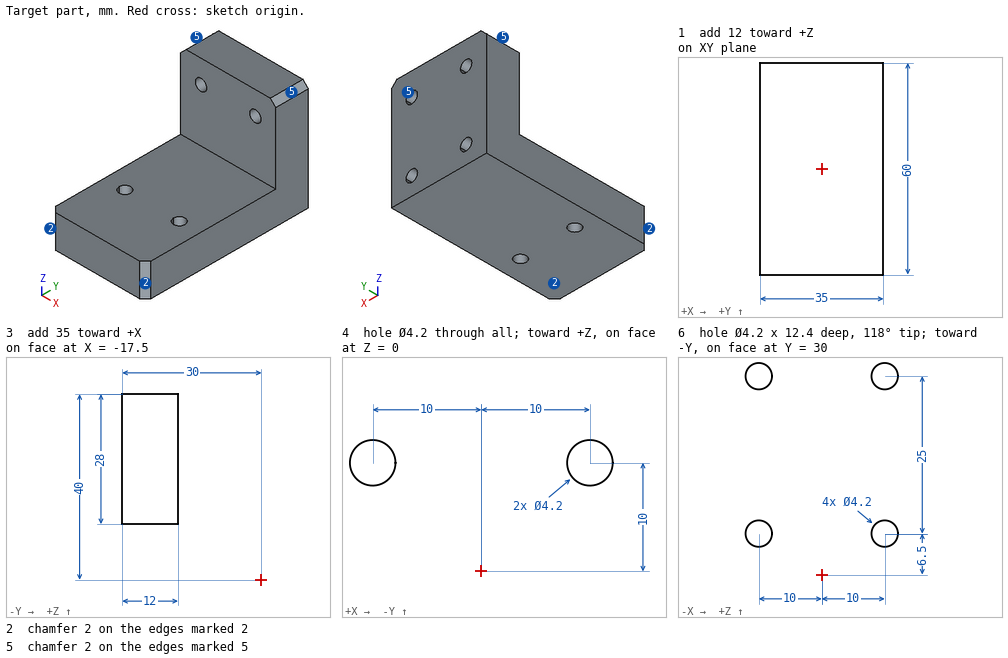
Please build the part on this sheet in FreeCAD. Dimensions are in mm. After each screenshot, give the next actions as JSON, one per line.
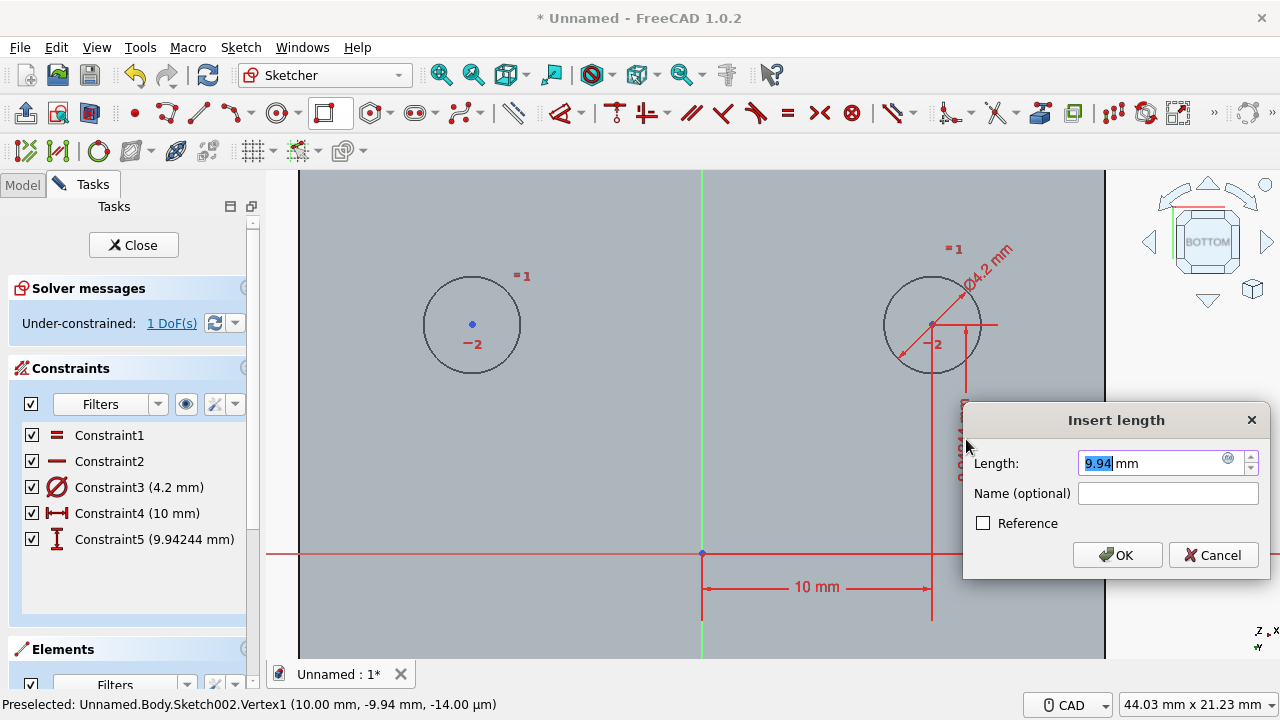
{"action": "type", "text": "10"}
{"action": "key", "text": "Return"}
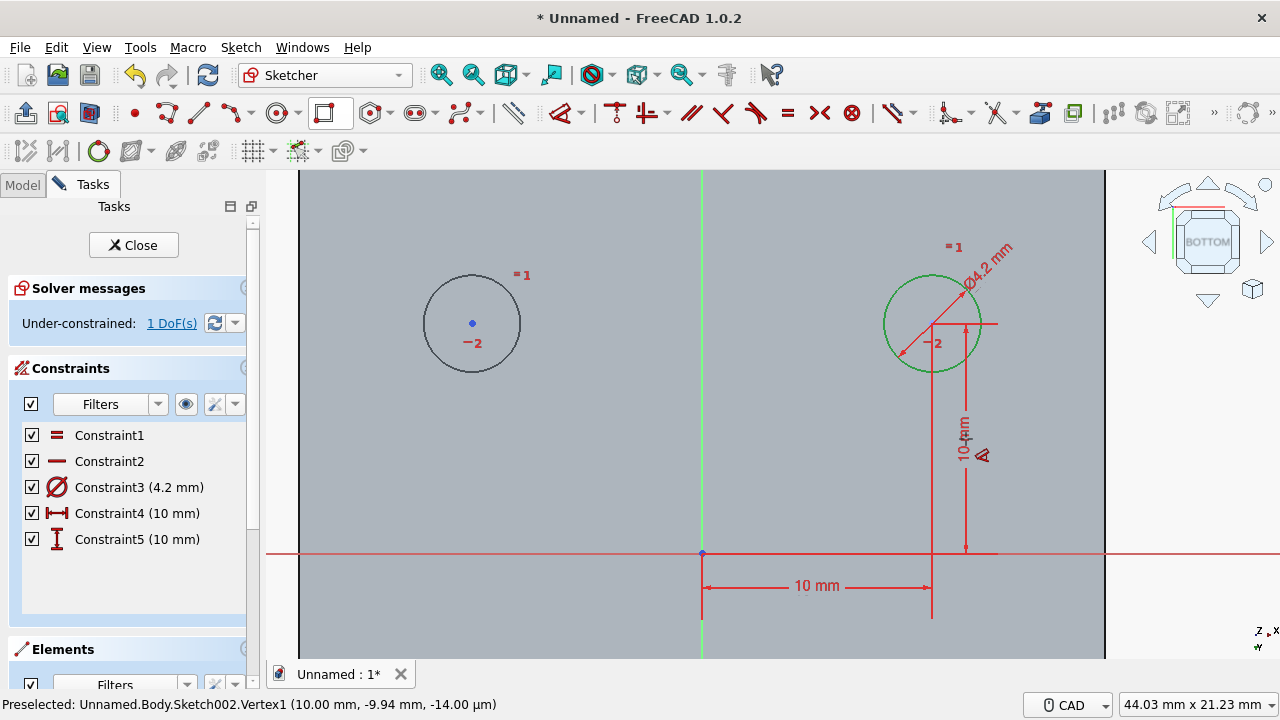
{"action": "left_click", "coordinate": [472, 324]}
{"action": "left_click", "coordinate": [587, 588]}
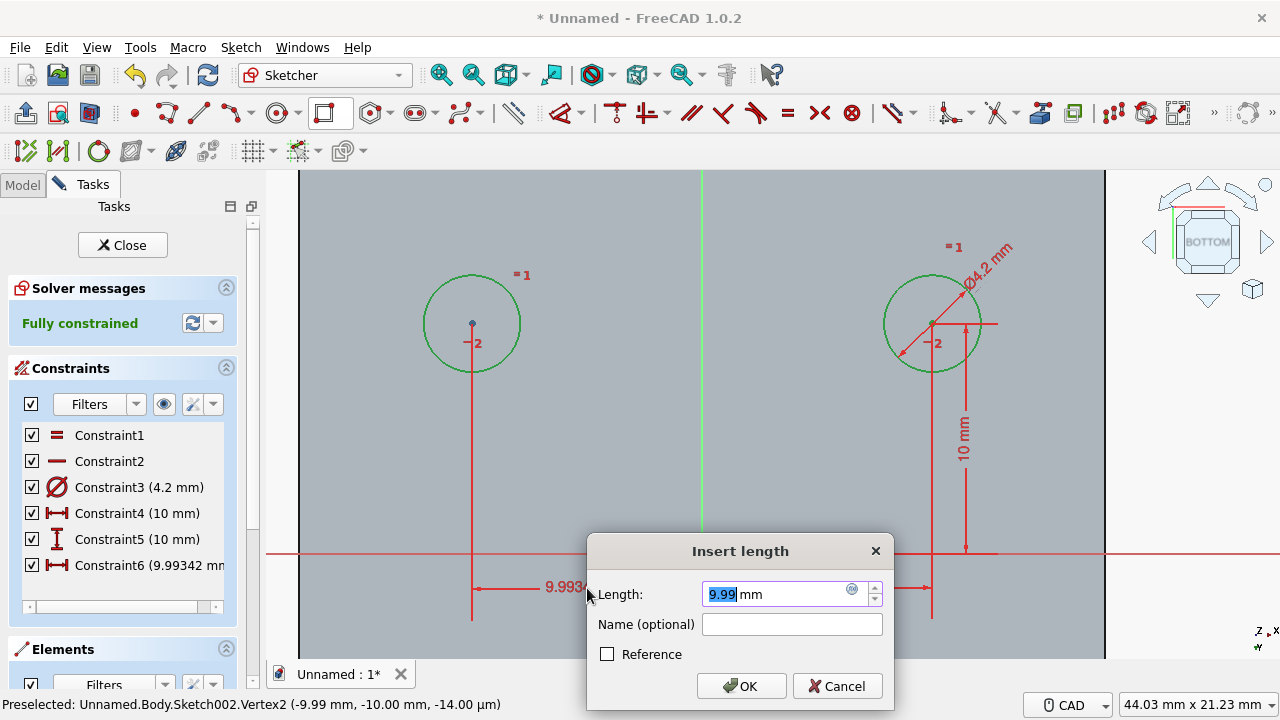
{"action": "type", "text": "10"}
{"action": "key", "text": "Return"}
{"action": "key", "text": "Escape"}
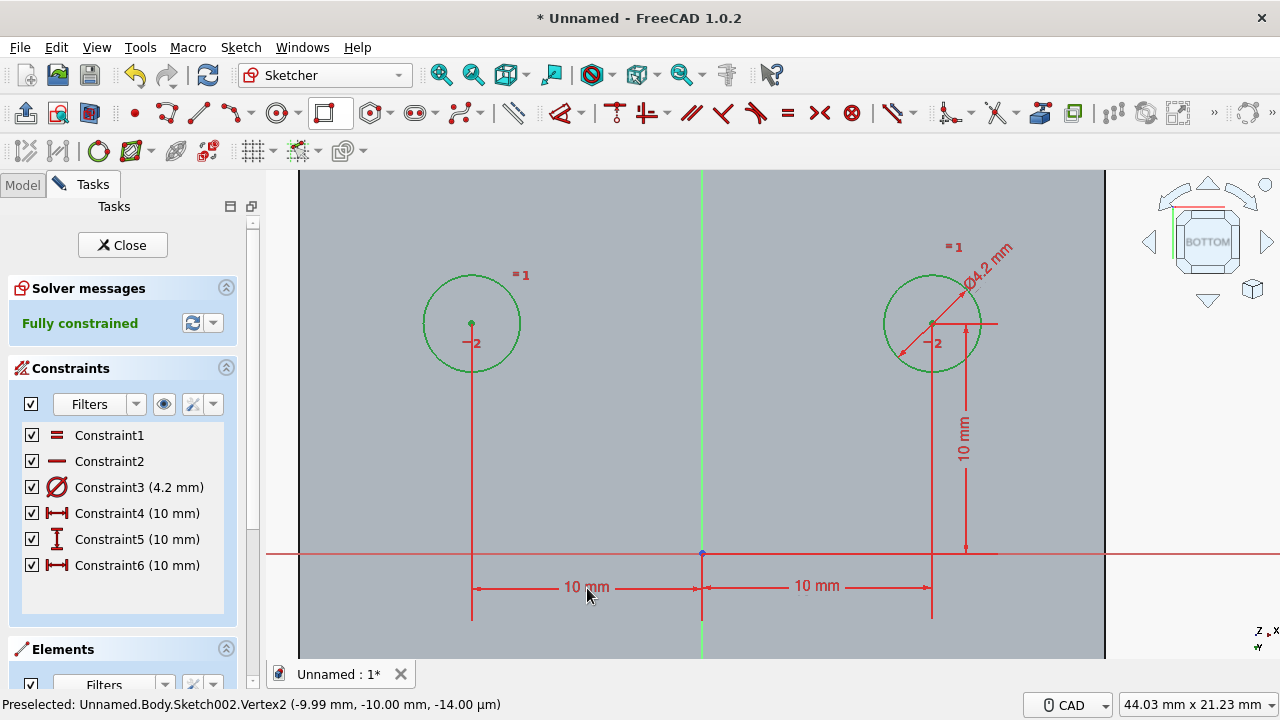
{"action": "left_click", "coordinate": [123, 245]}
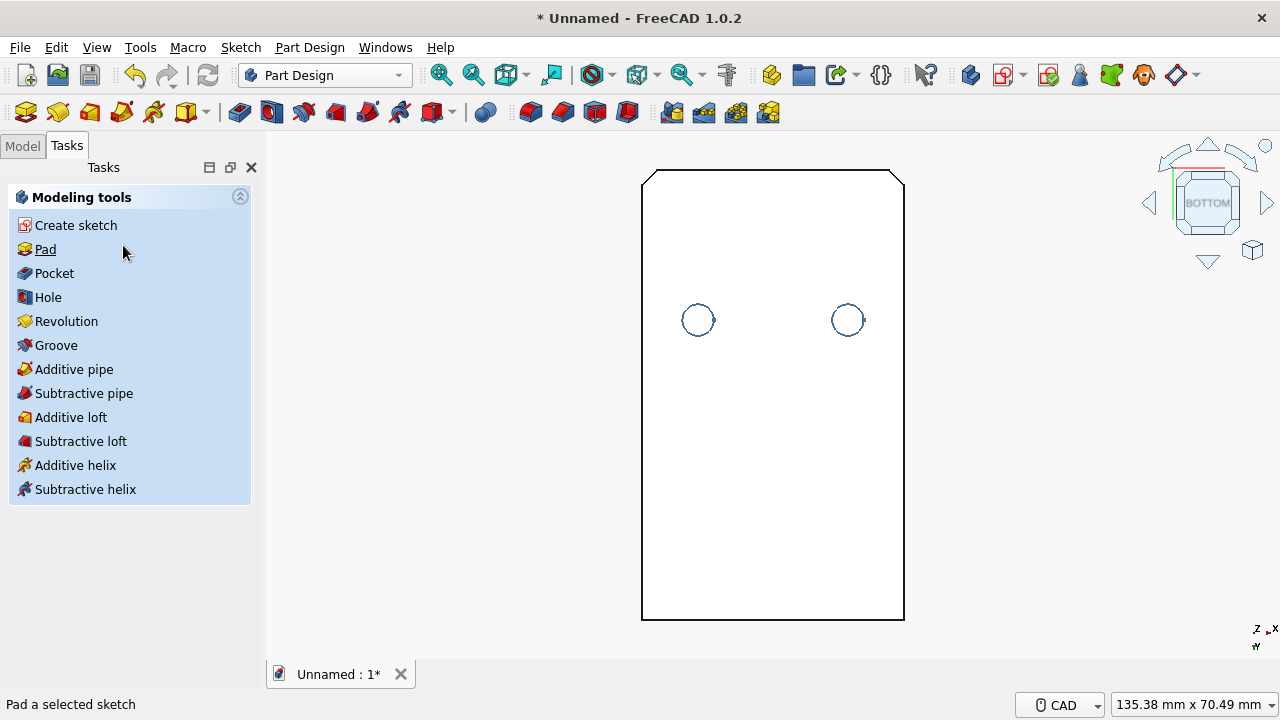
{"action": "left_click", "coordinate": [272, 112]}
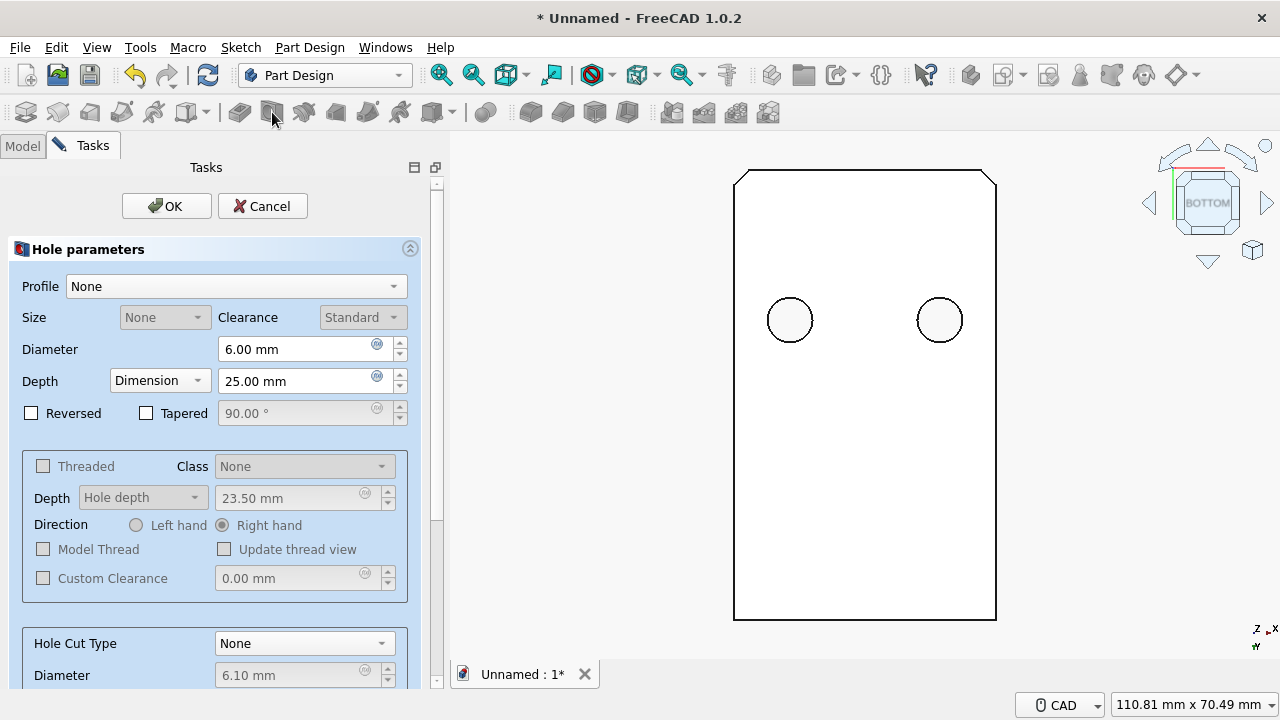
{"action": "triple_click", "coordinate": [305, 349]}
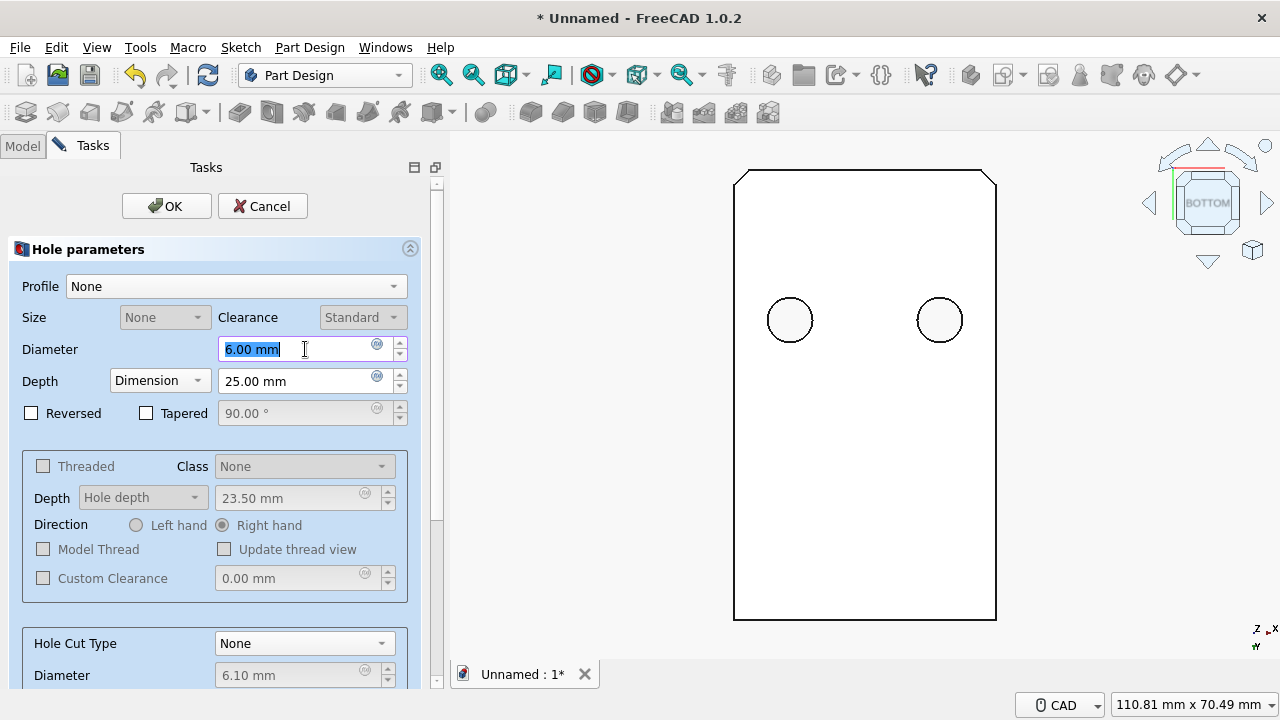
{"action": "type", "text": "4.2"}
{"action": "key", "text": "Tab"}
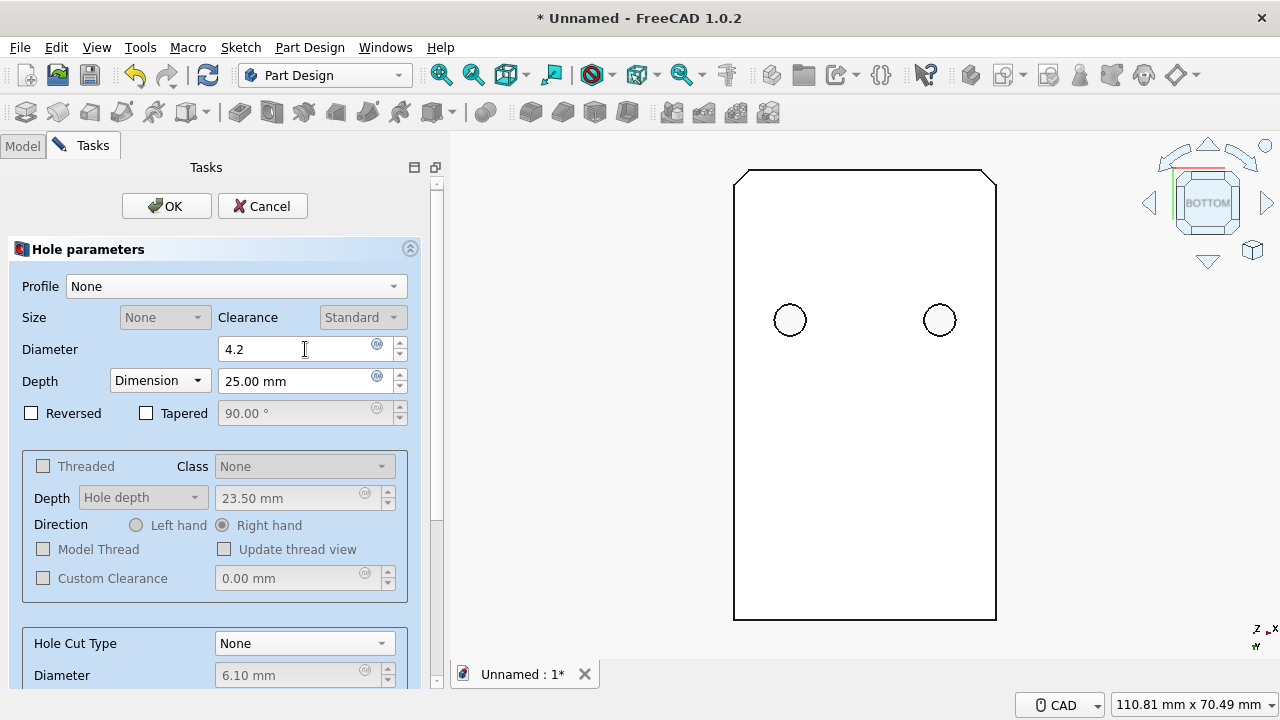
{"action": "left_click", "coordinate": [161, 380]}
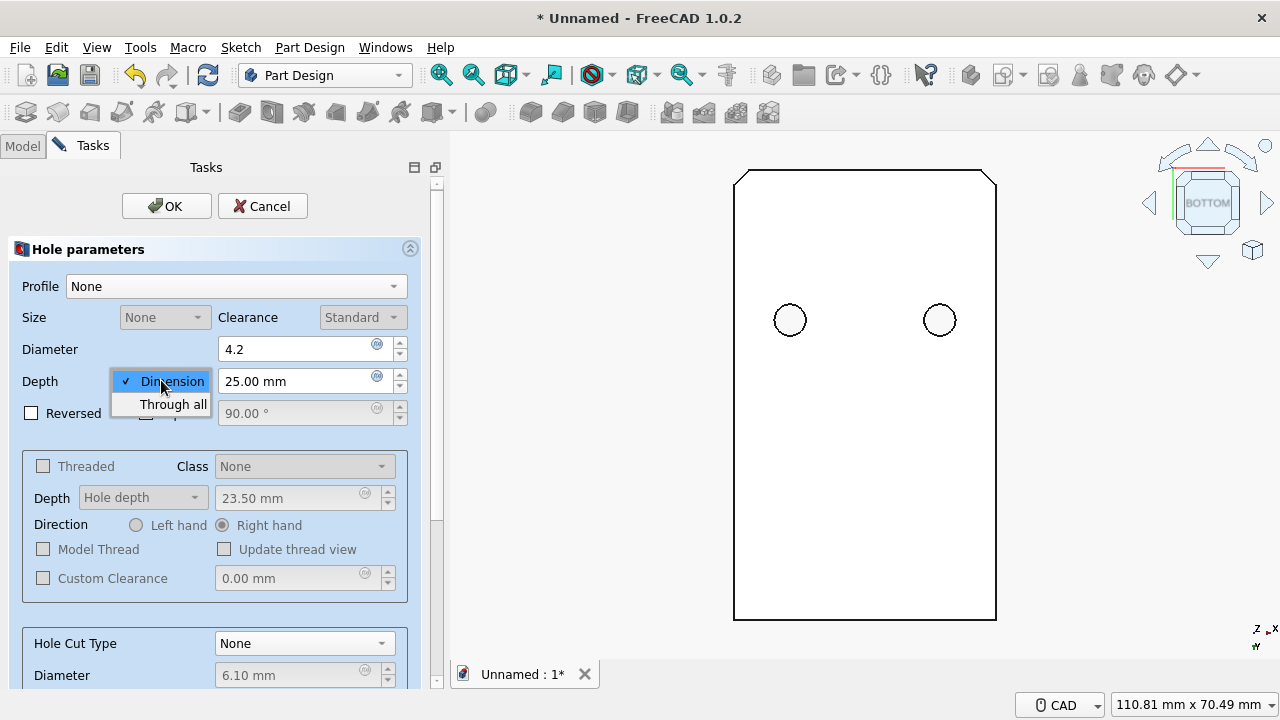
{"action": "left_click", "coordinate": [160, 404]}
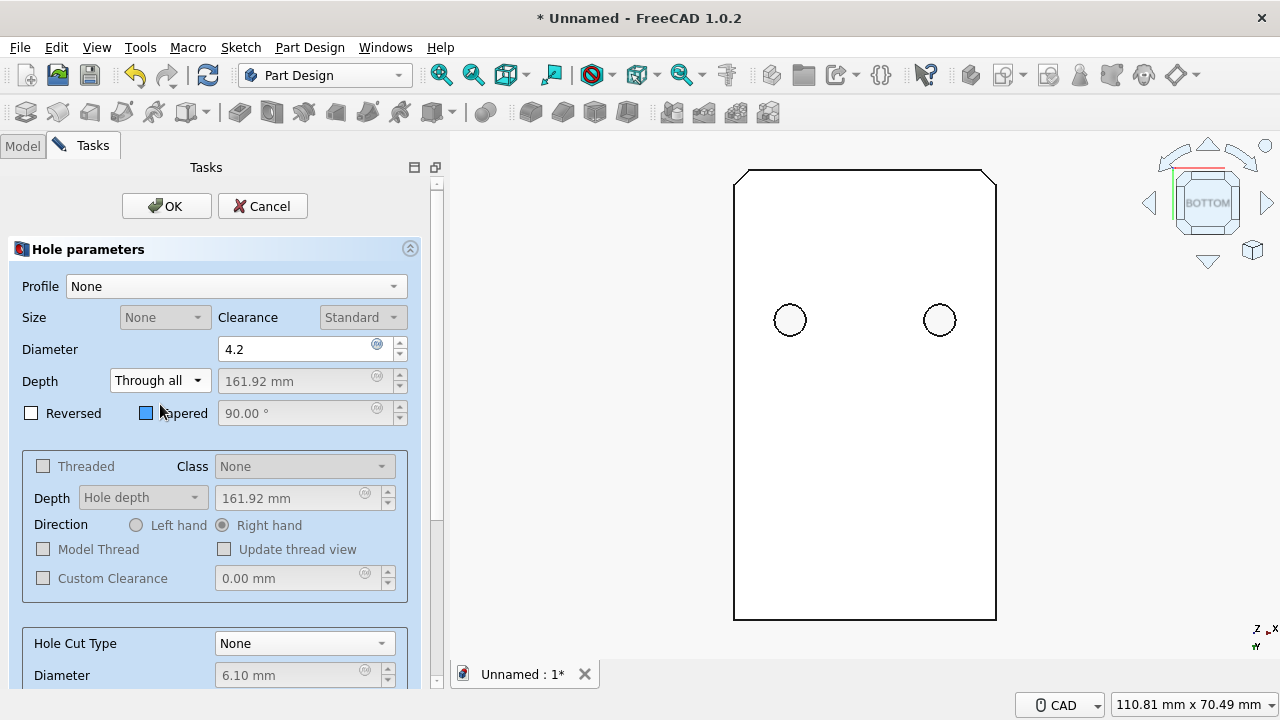
{"action": "left_click", "coordinate": [167, 206]}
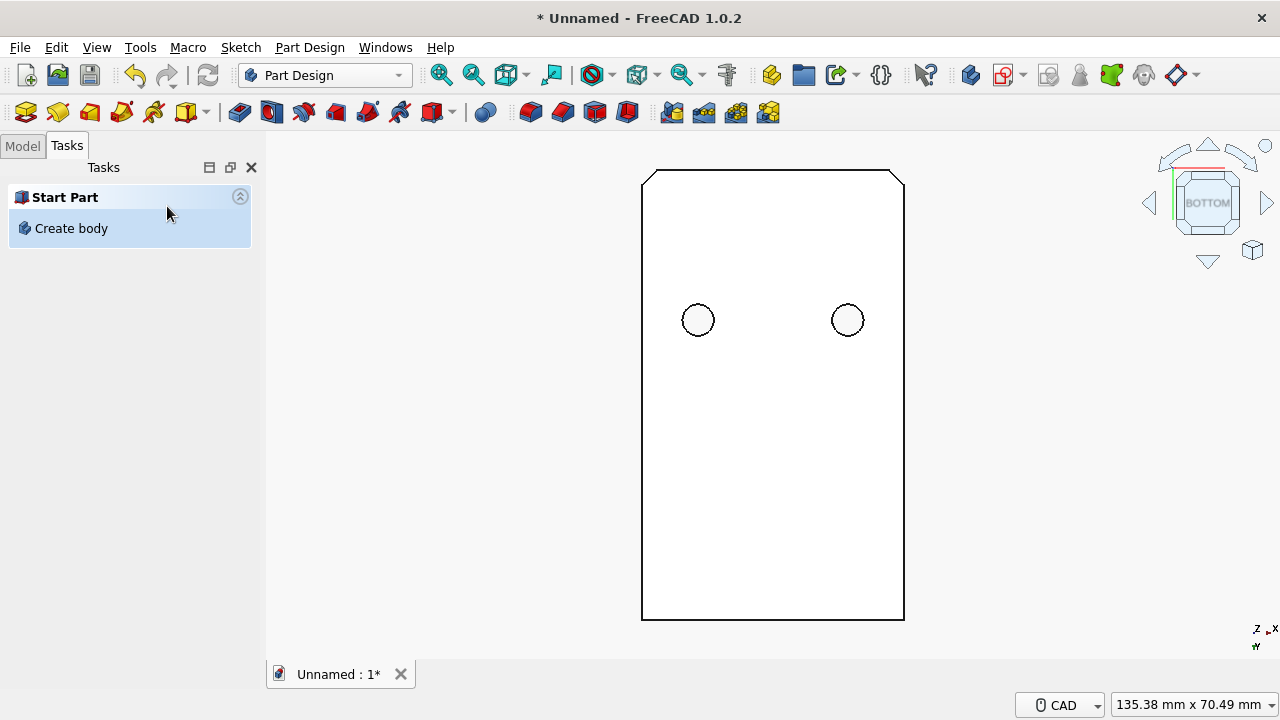
{"action": "key", "text": "0"}